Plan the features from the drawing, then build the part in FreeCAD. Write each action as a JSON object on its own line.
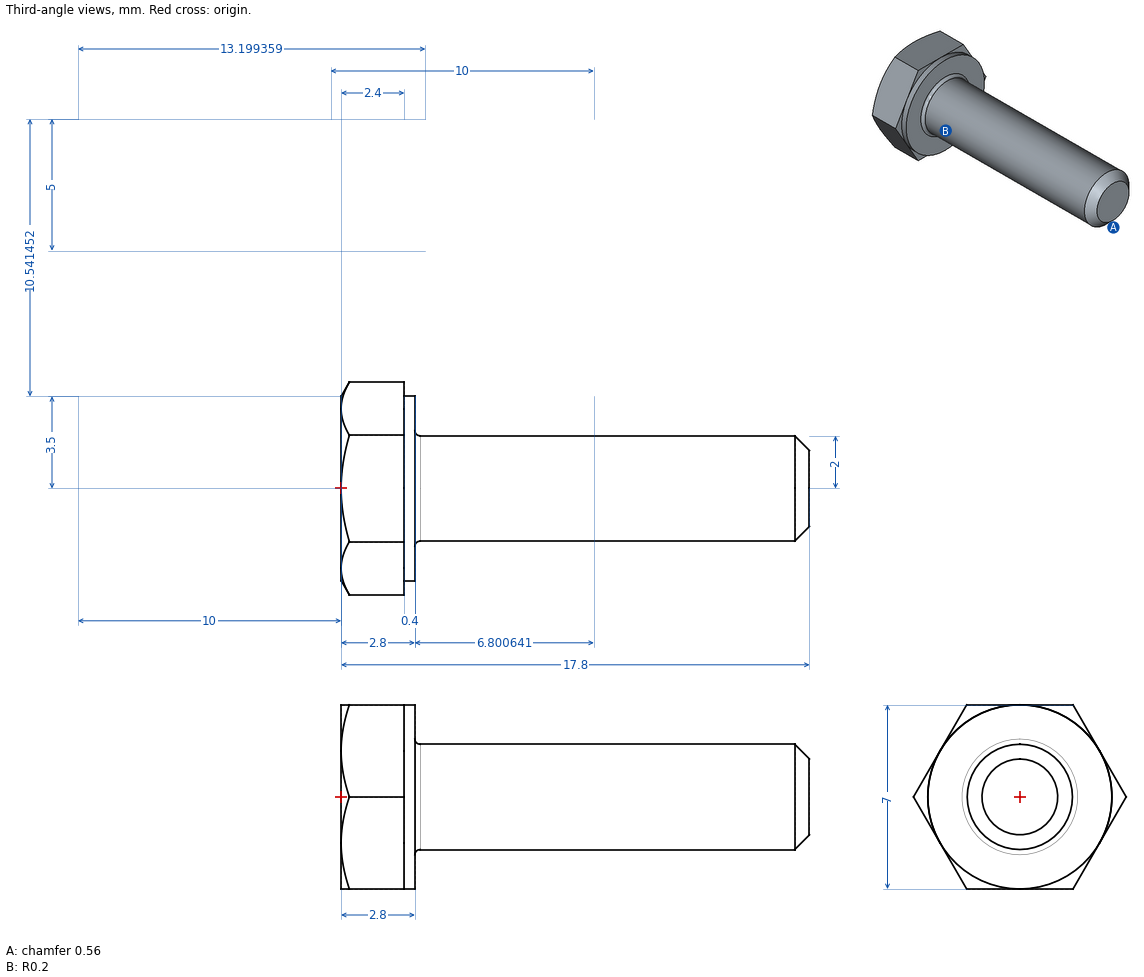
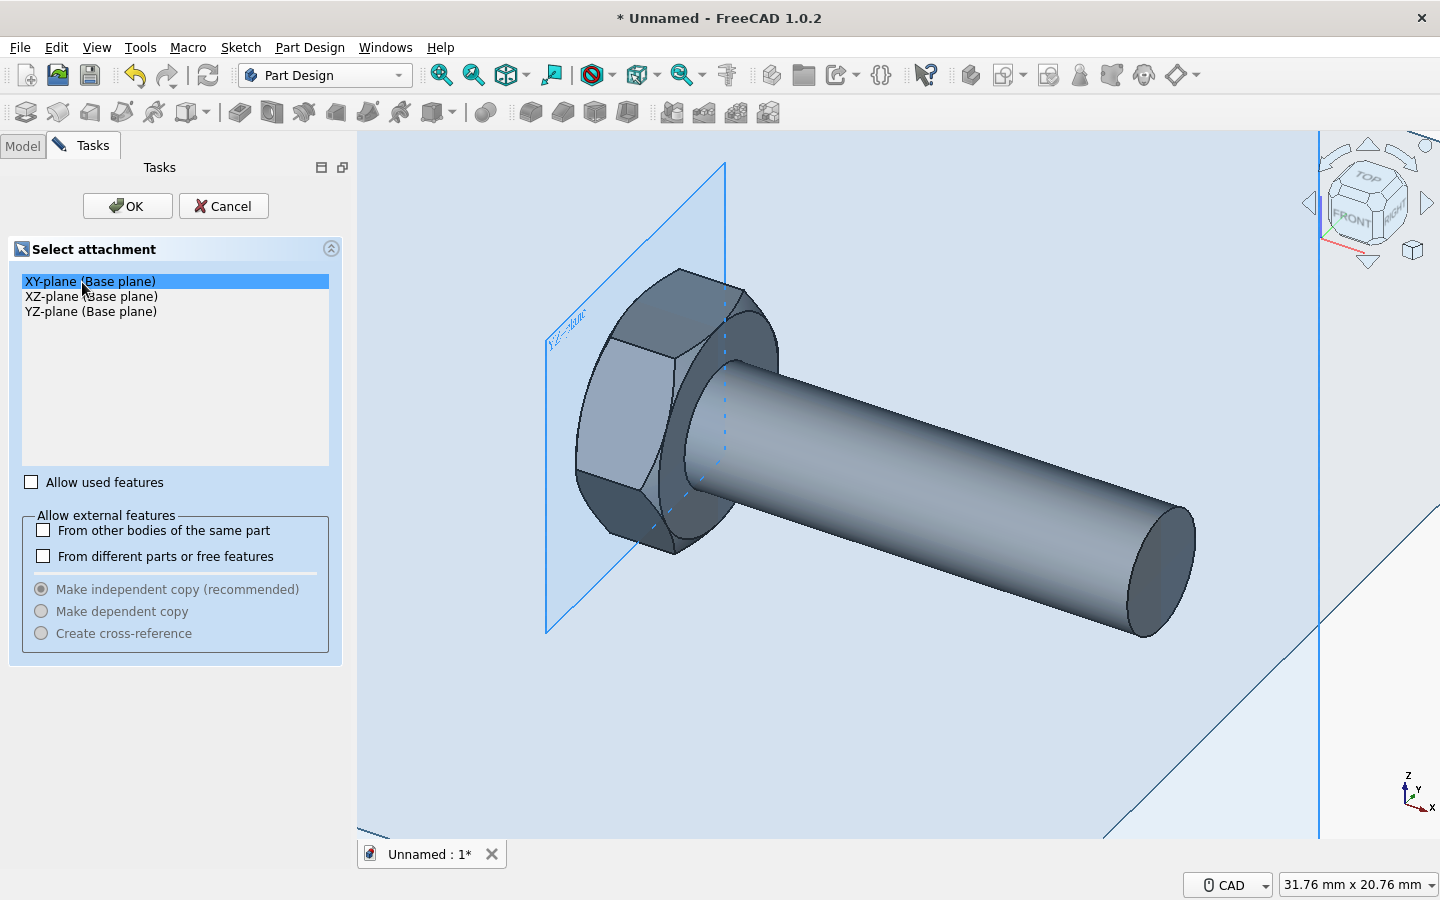
{"action": "left_click", "coordinate": [128, 206]}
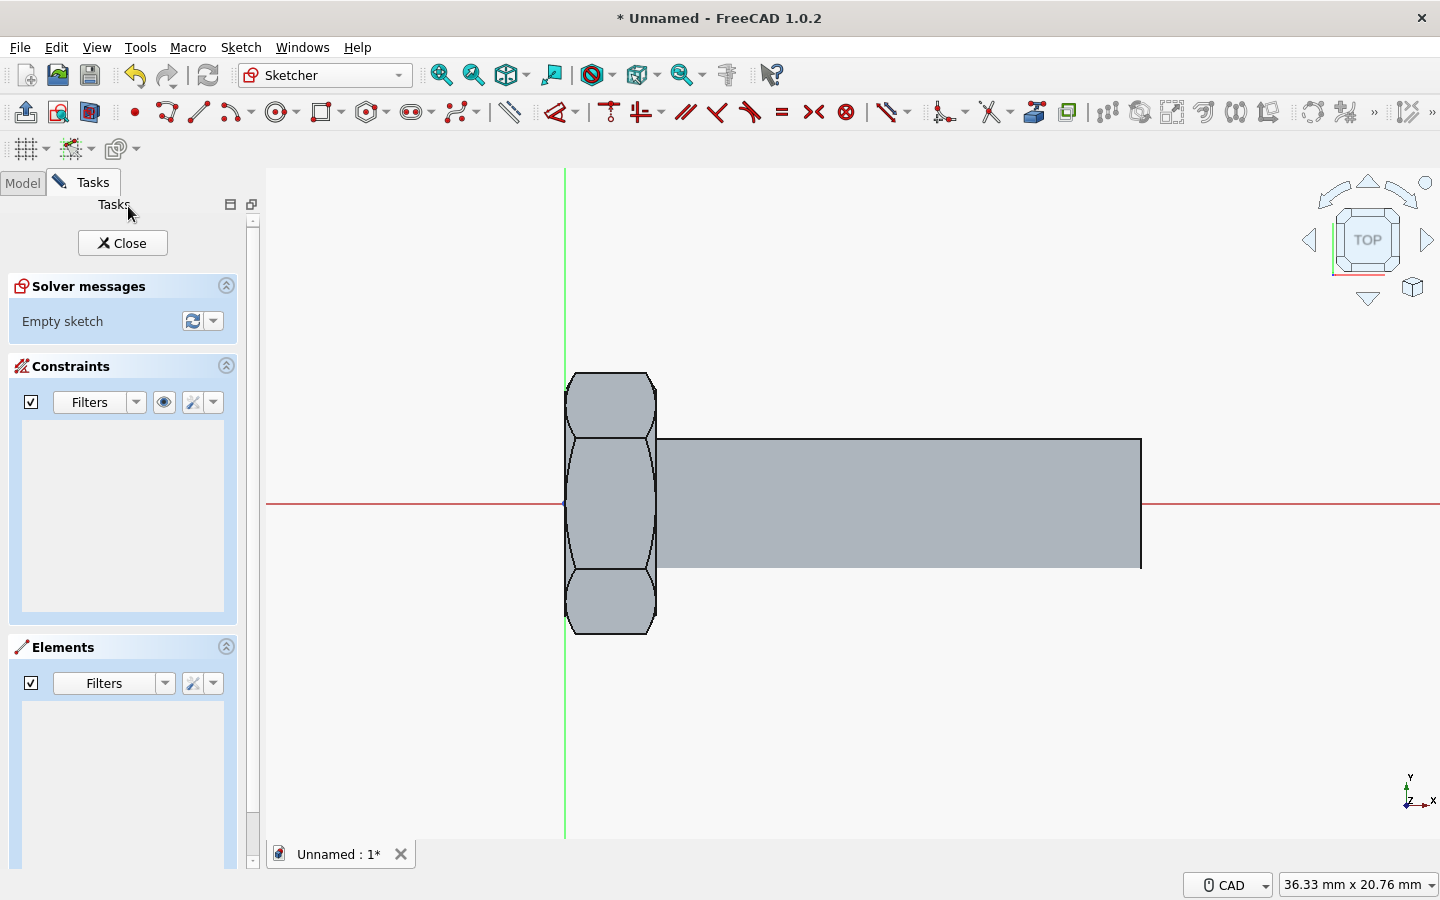
{"action": "left_click", "coordinate": [90, 112]}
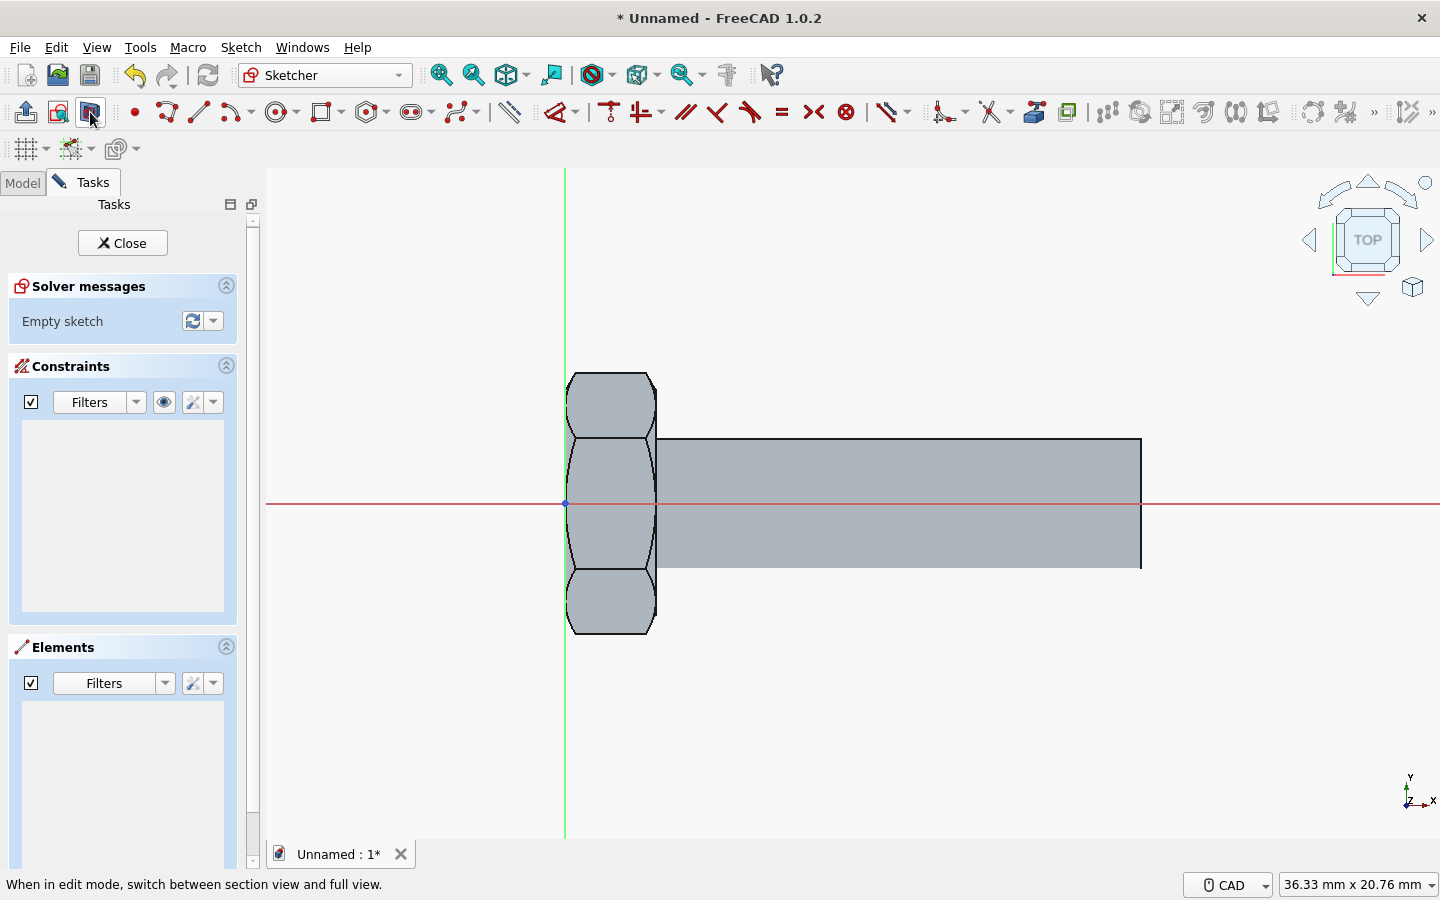
{"action": "scroll", "coordinate": [1138, 811], "scroll_direction": "down", "scroll_amount": 2}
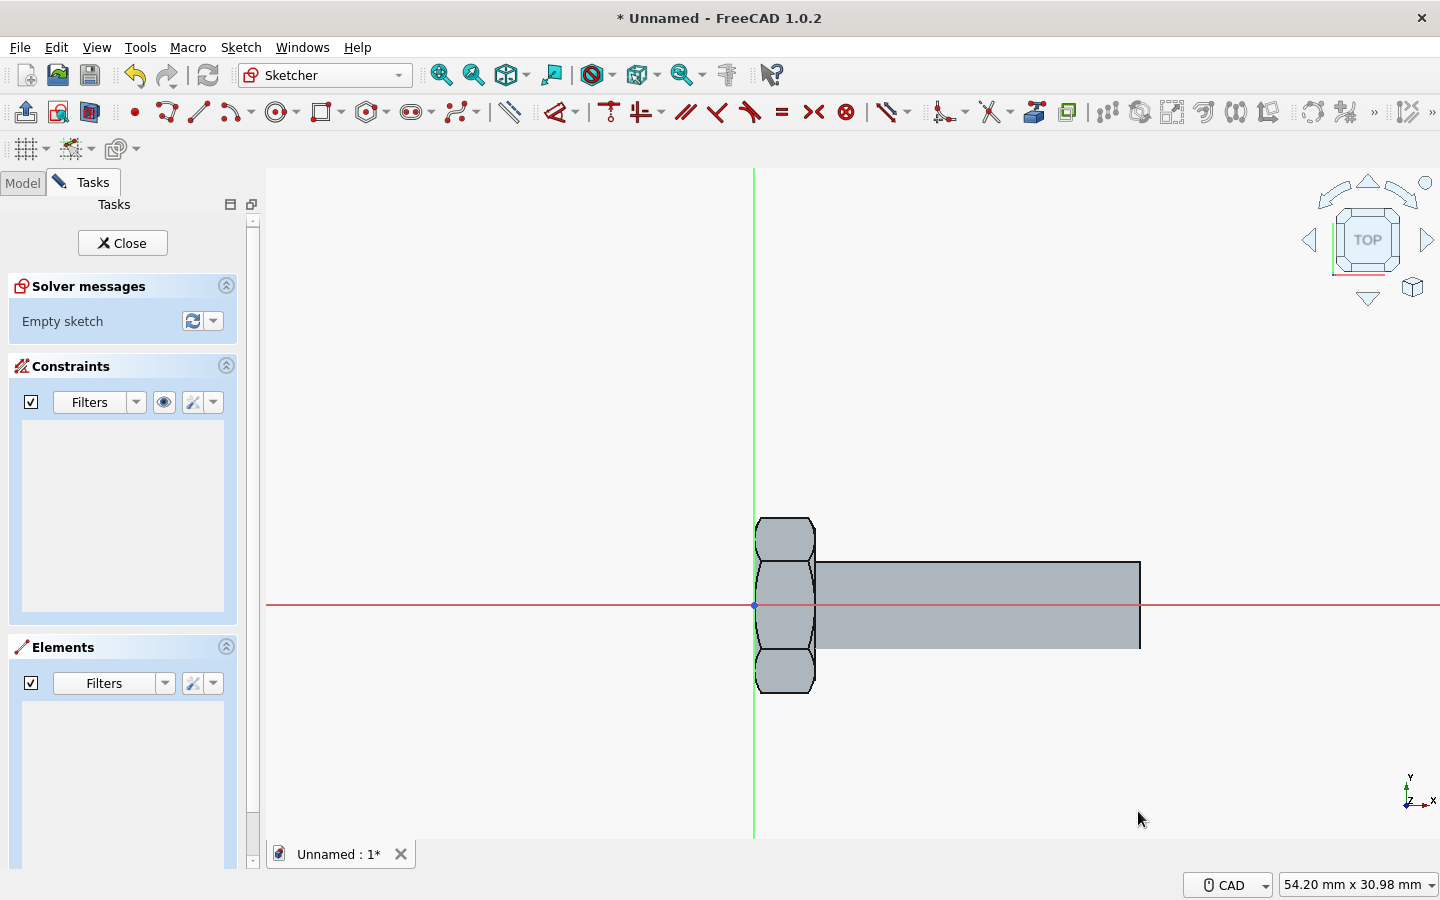
{"action": "scroll", "coordinate": [785, 351], "scroll_direction": "up", "scroll_amount": 2}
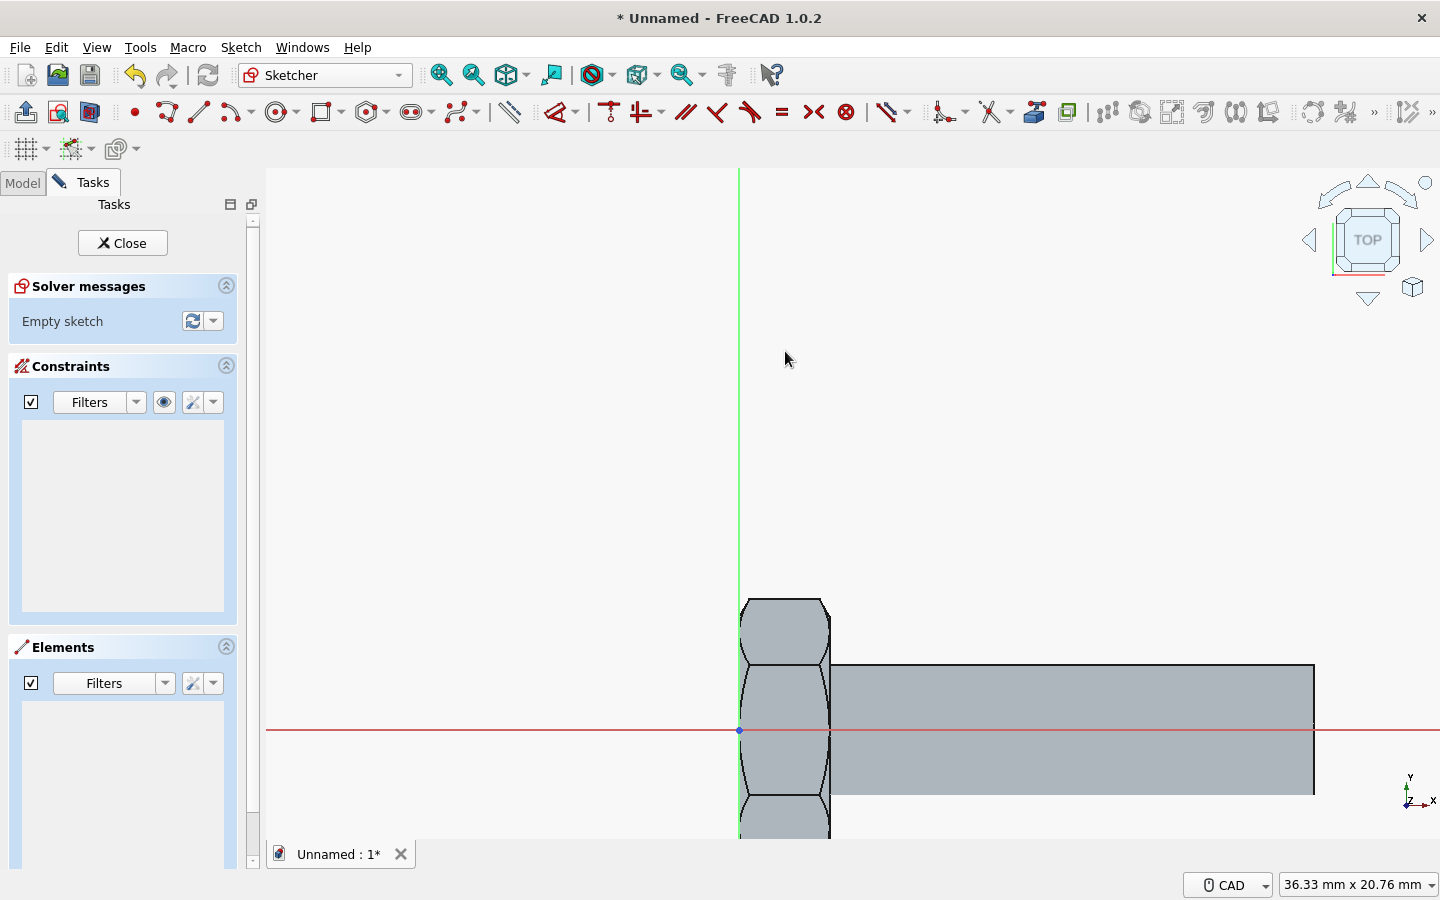
{"action": "key", "text": "g r"}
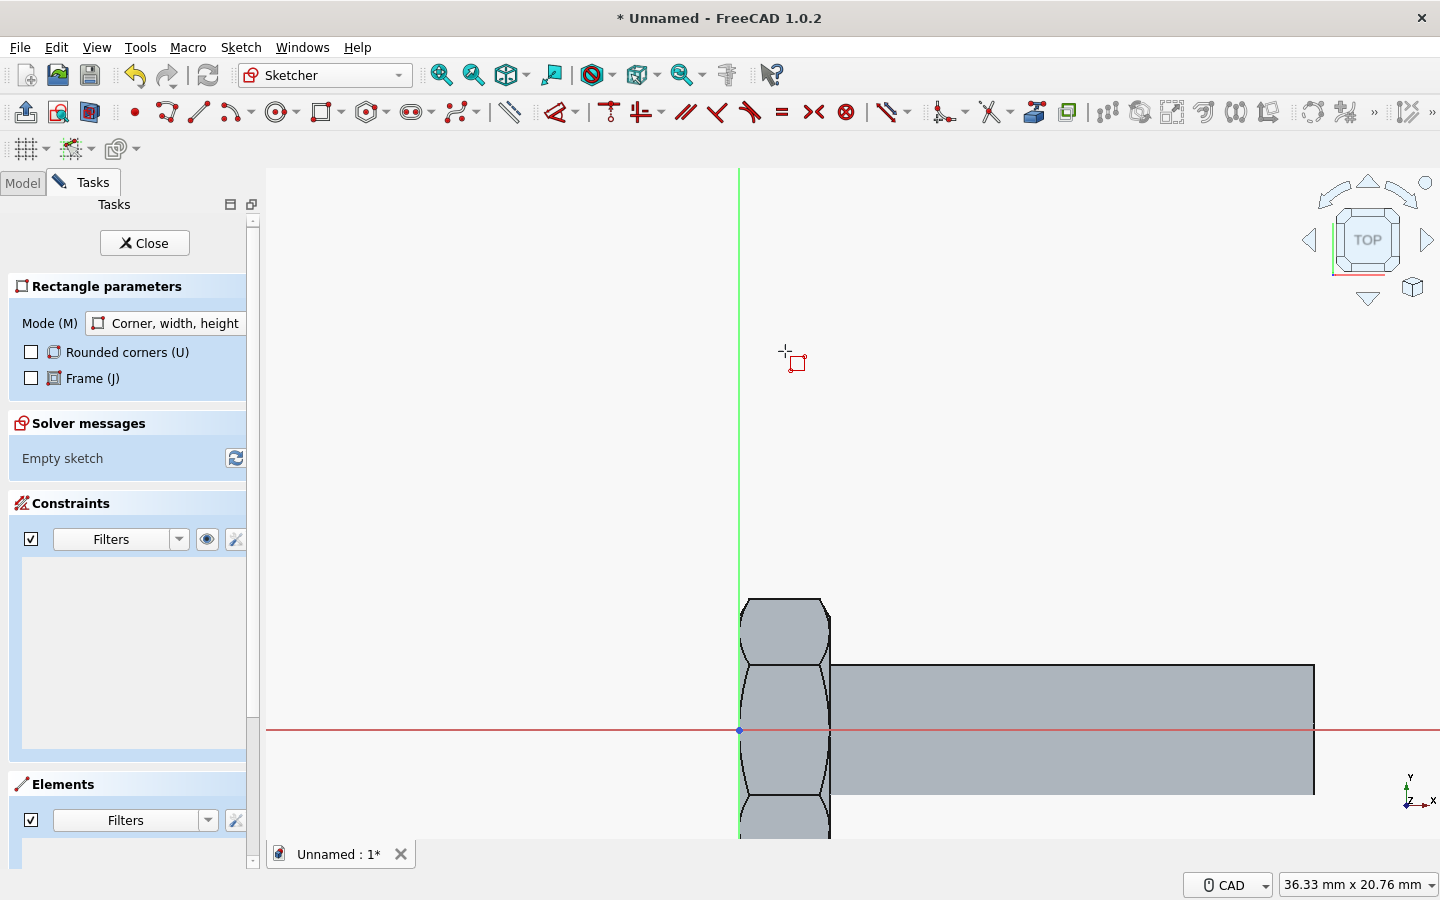
{"action": "scroll", "coordinate": [817, 276], "scroll_direction": "up", "scroll_amount": 2}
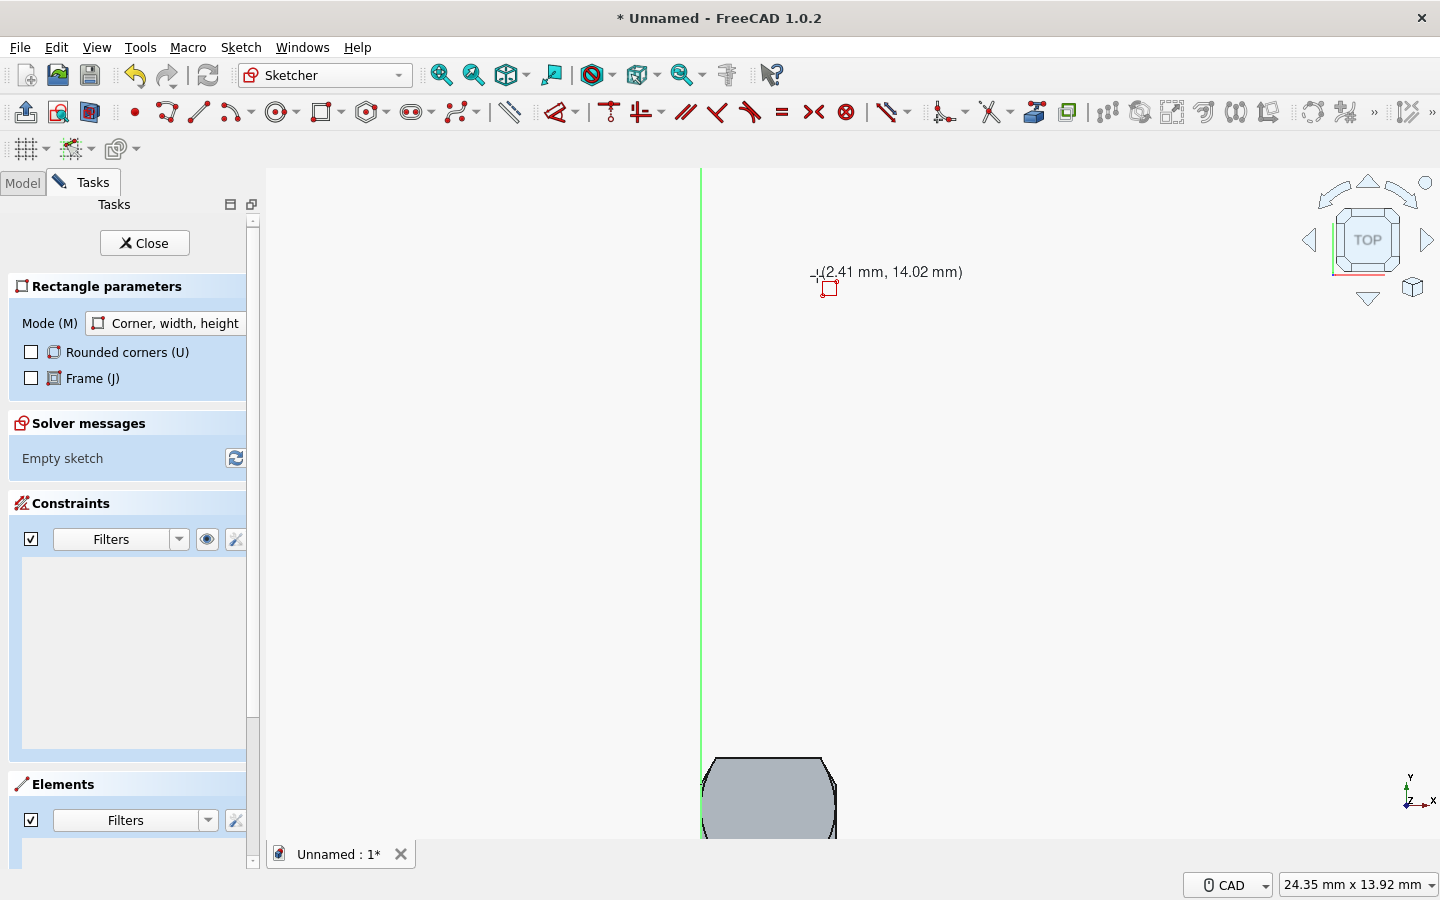
{"action": "left_click", "coordinate": [816, 276]}
{"action": "left_click", "coordinate": [836, 785]}
{"action": "key", "text": "Escape"}